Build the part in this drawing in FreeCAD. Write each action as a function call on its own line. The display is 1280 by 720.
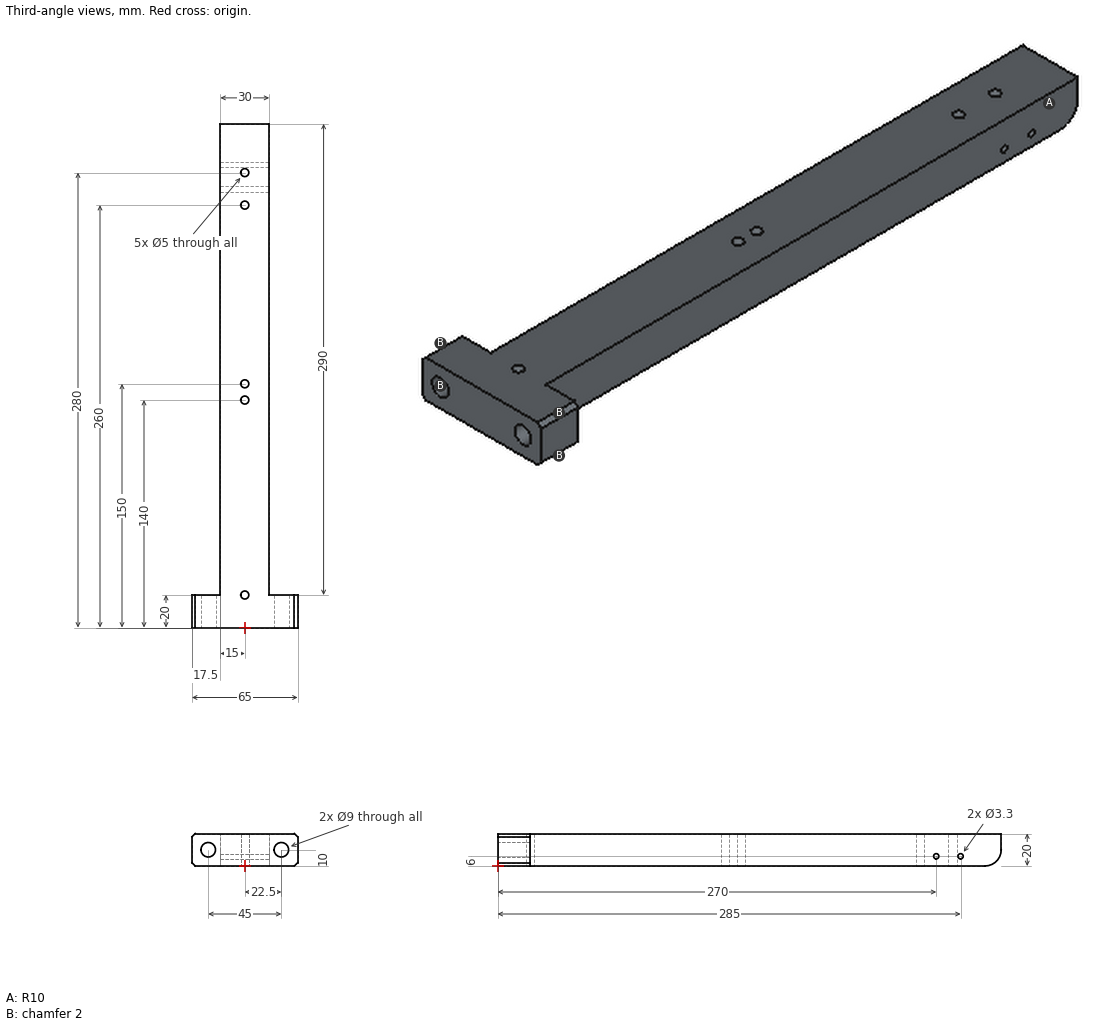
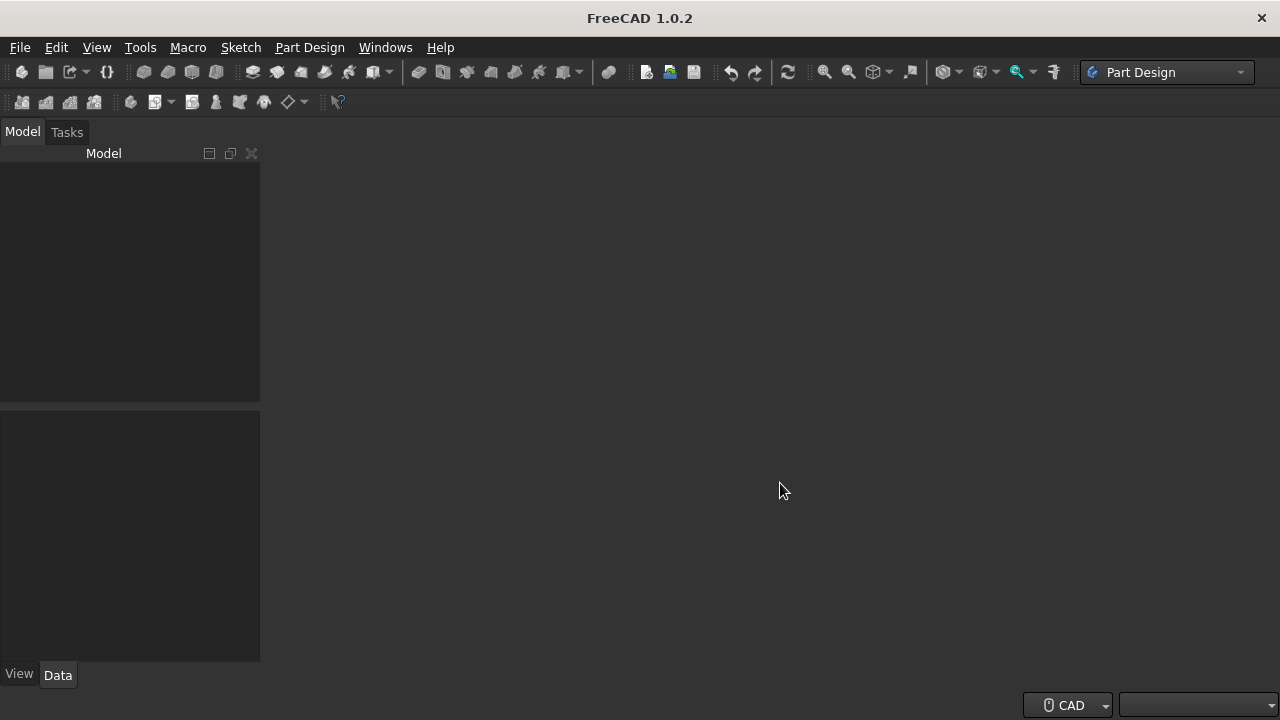
click(646, 72)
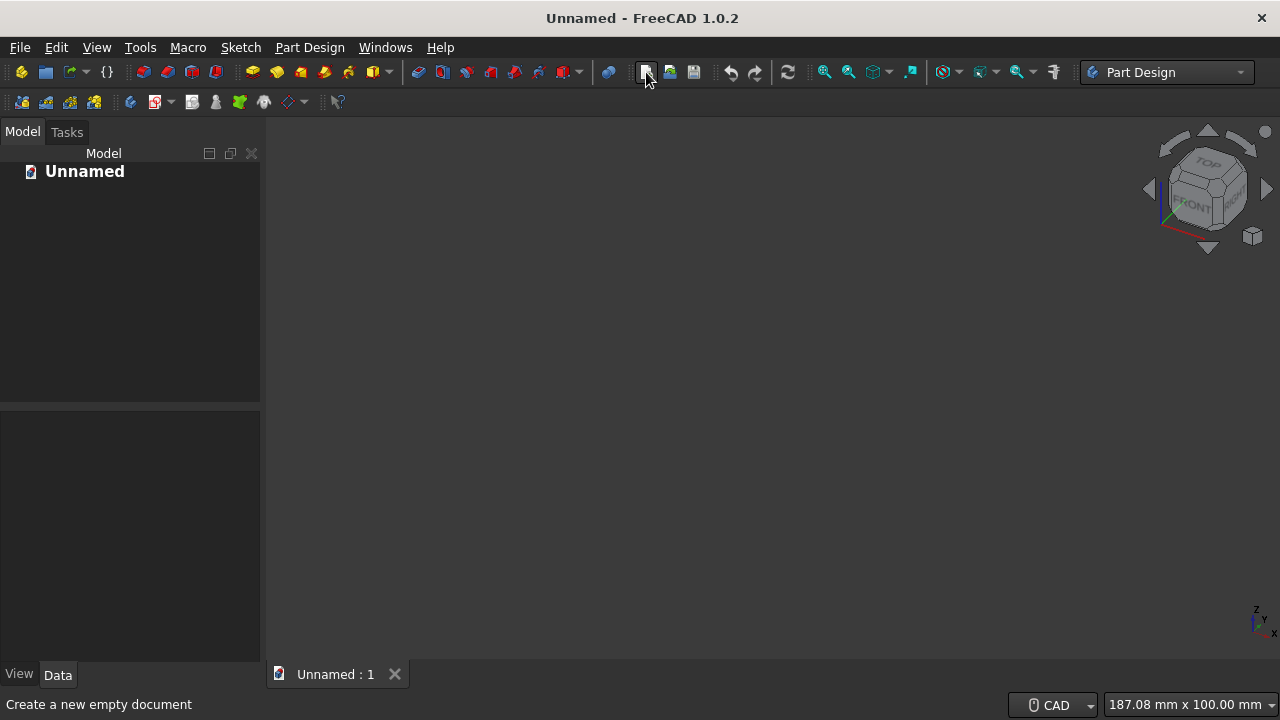
click(156, 102)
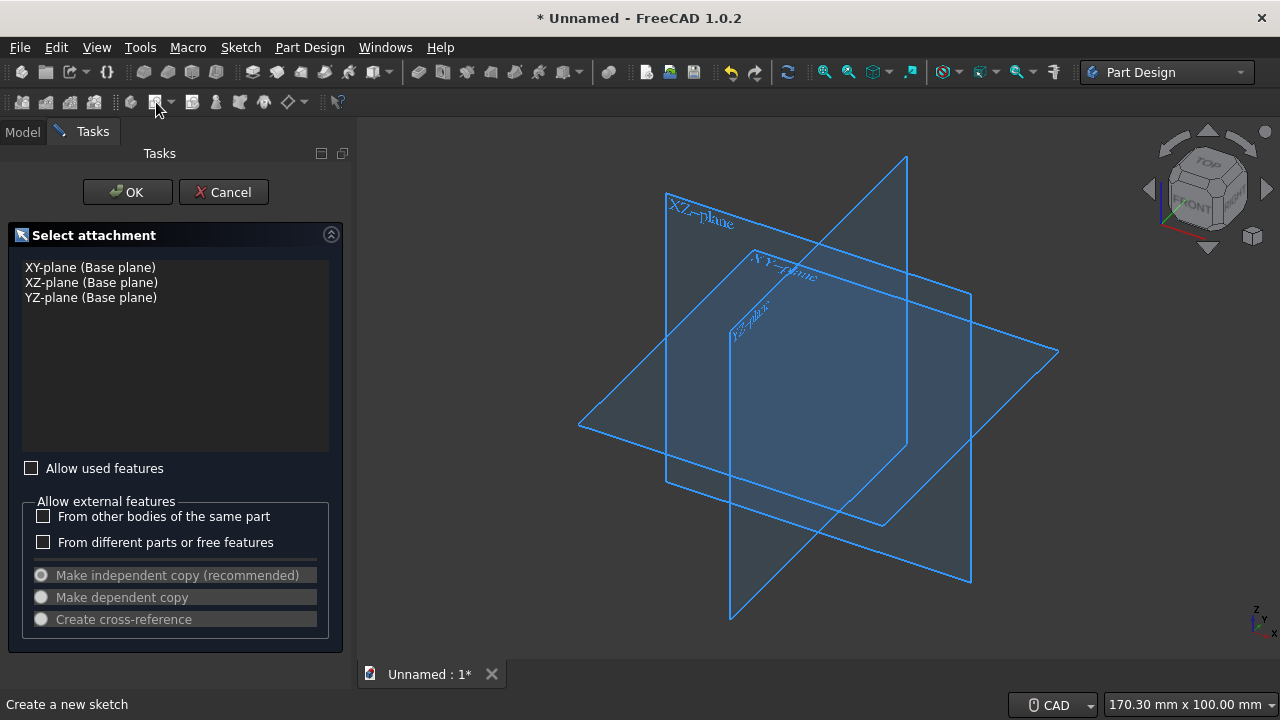
click(82, 268)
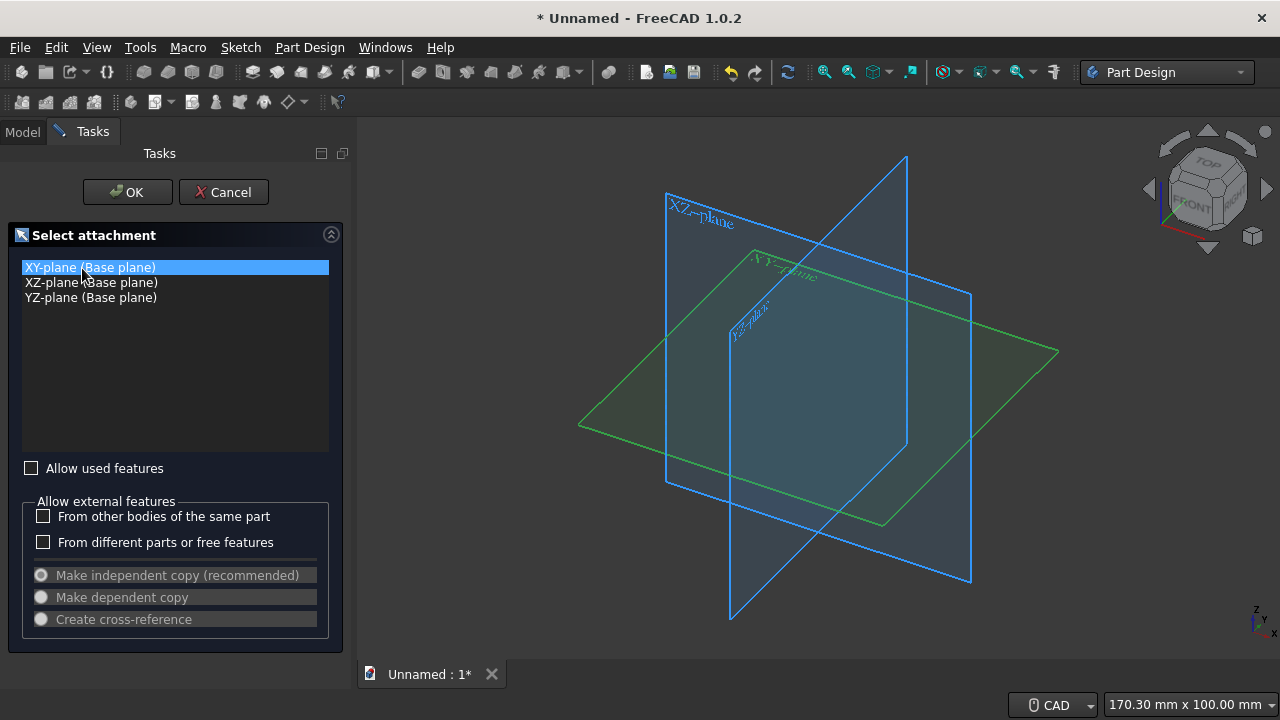
click(128, 192)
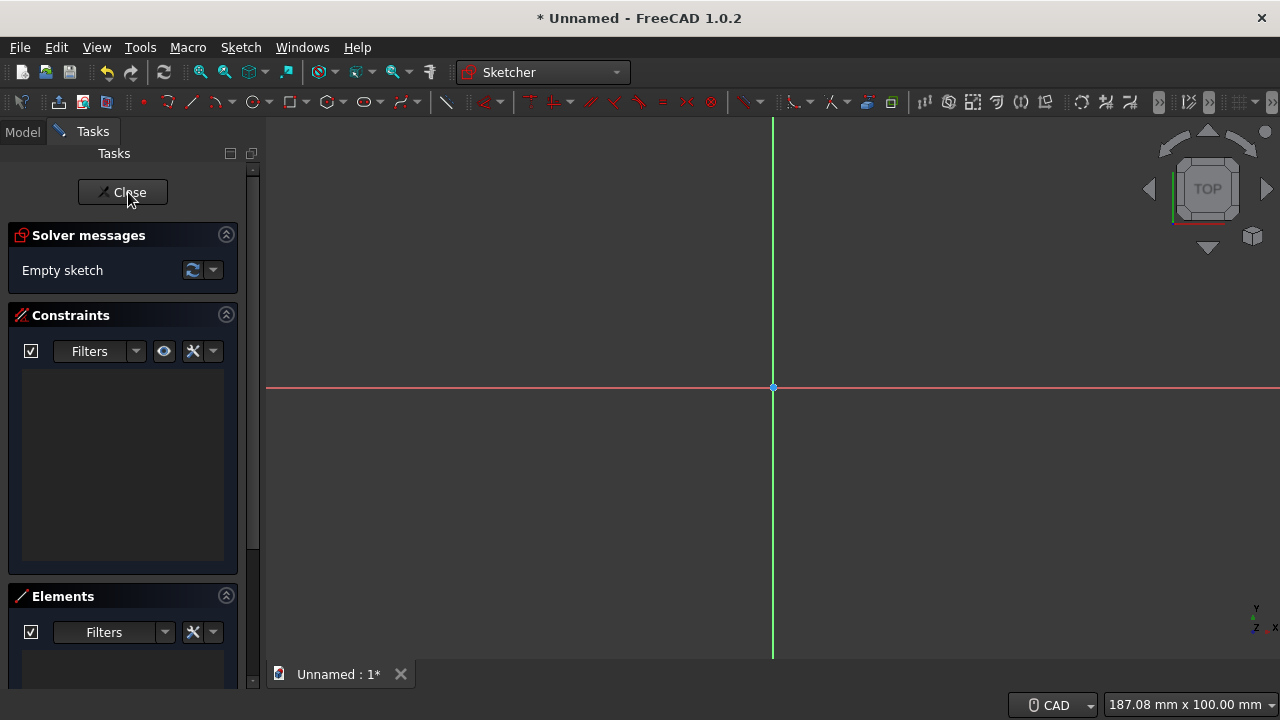
scroll(687, 601, down, 8)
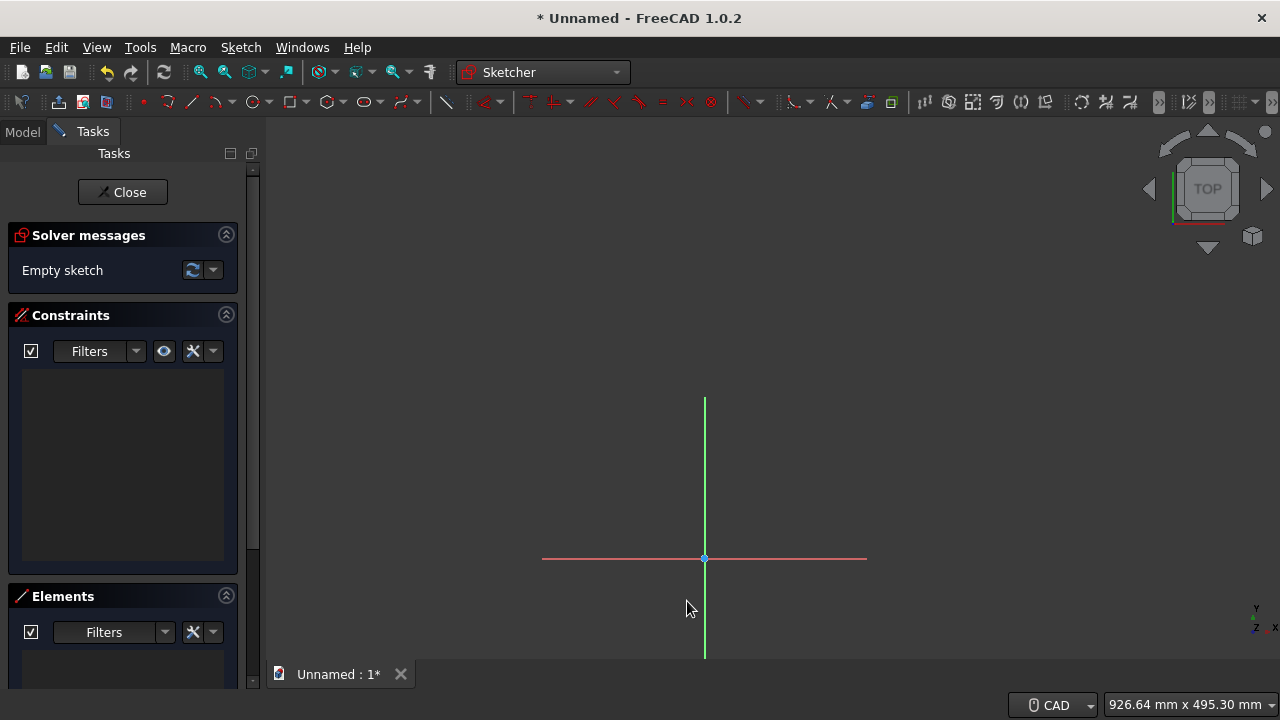
key(g)
key(m)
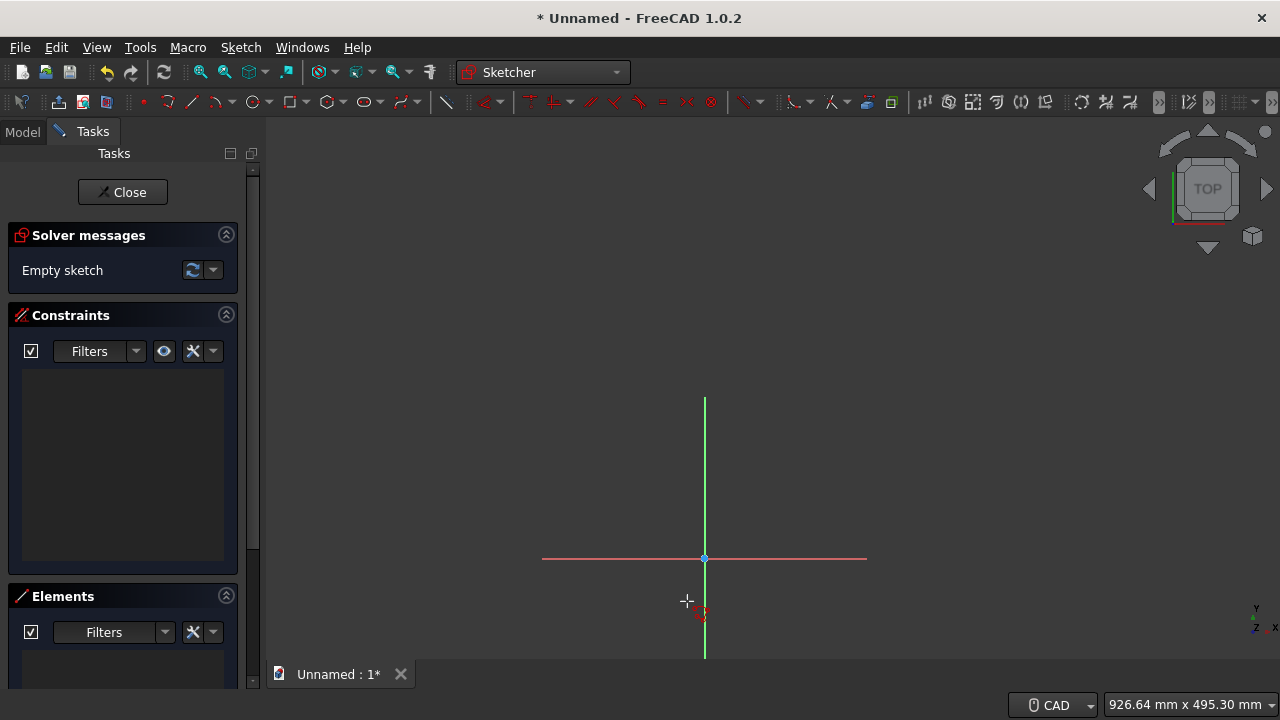
click(688, 537)
click(669, 537)
click(669, 559)
click(740, 550)
click(740, 537)
click(721, 537)
click(721, 219)
click(688, 219)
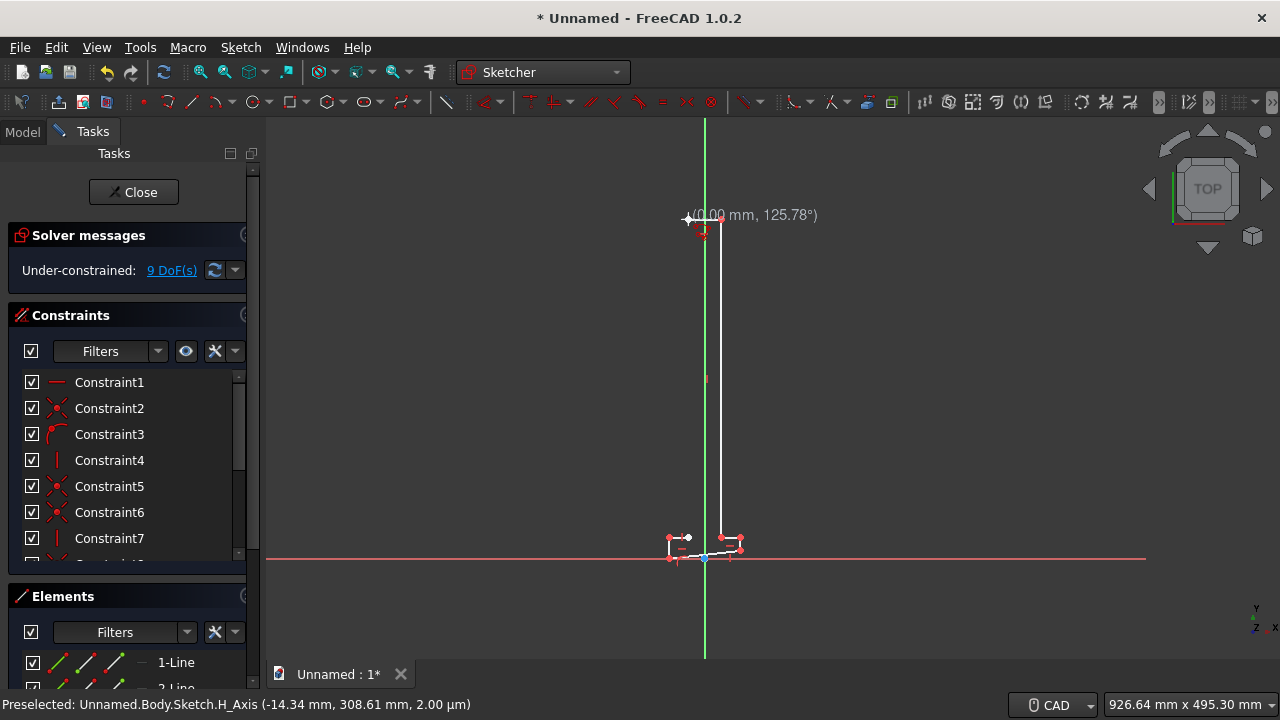
scroll(688, 537, up, 3)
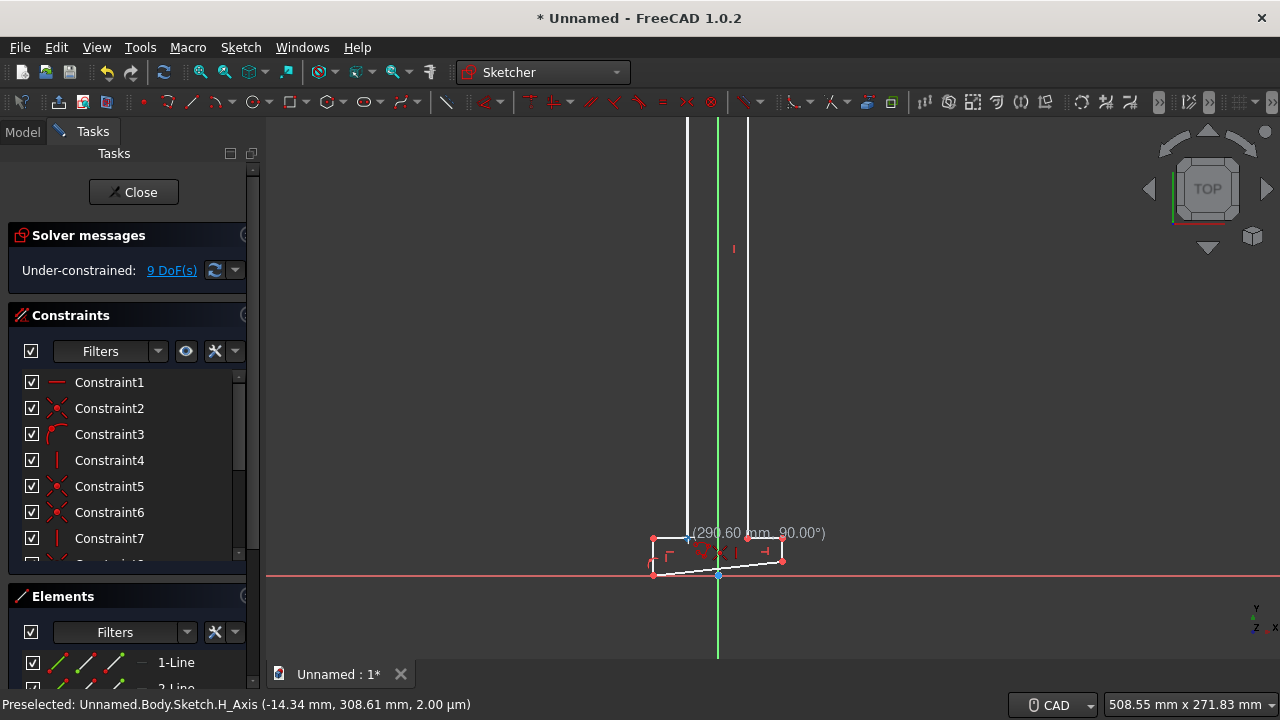
click(688, 538)
key(Escape)
key(Escape)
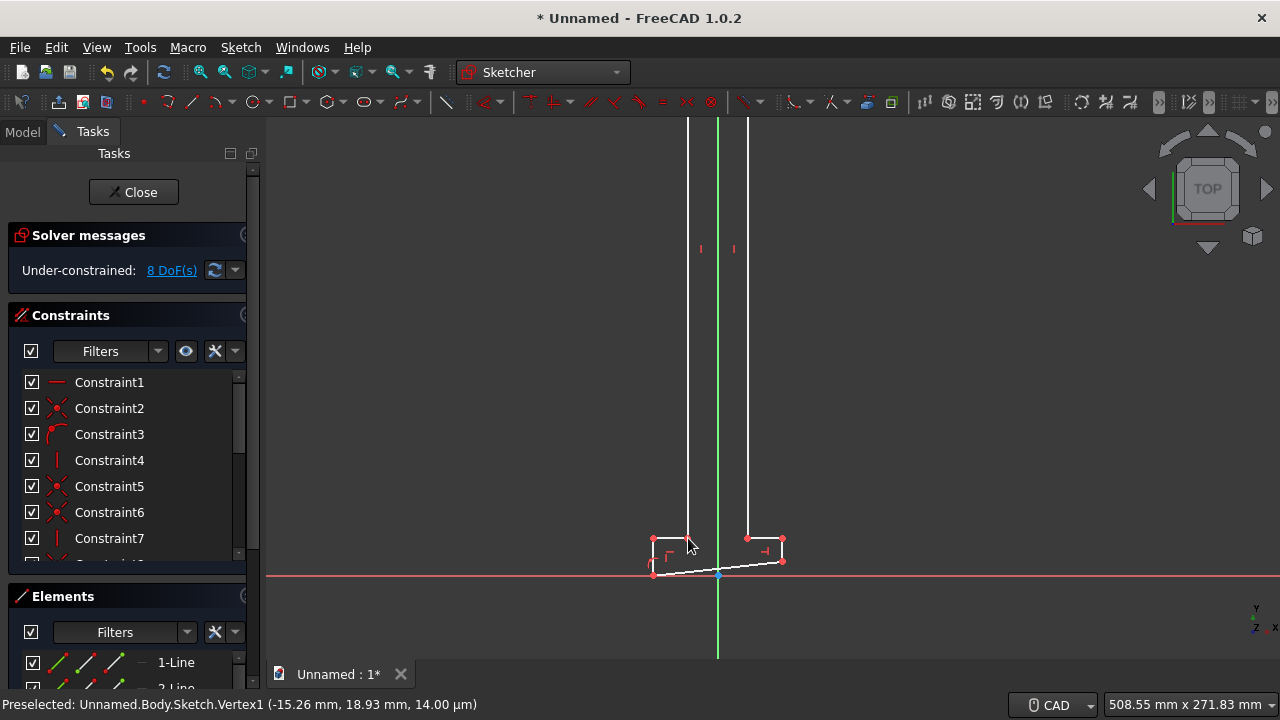
scroll(744, 566, up, 2)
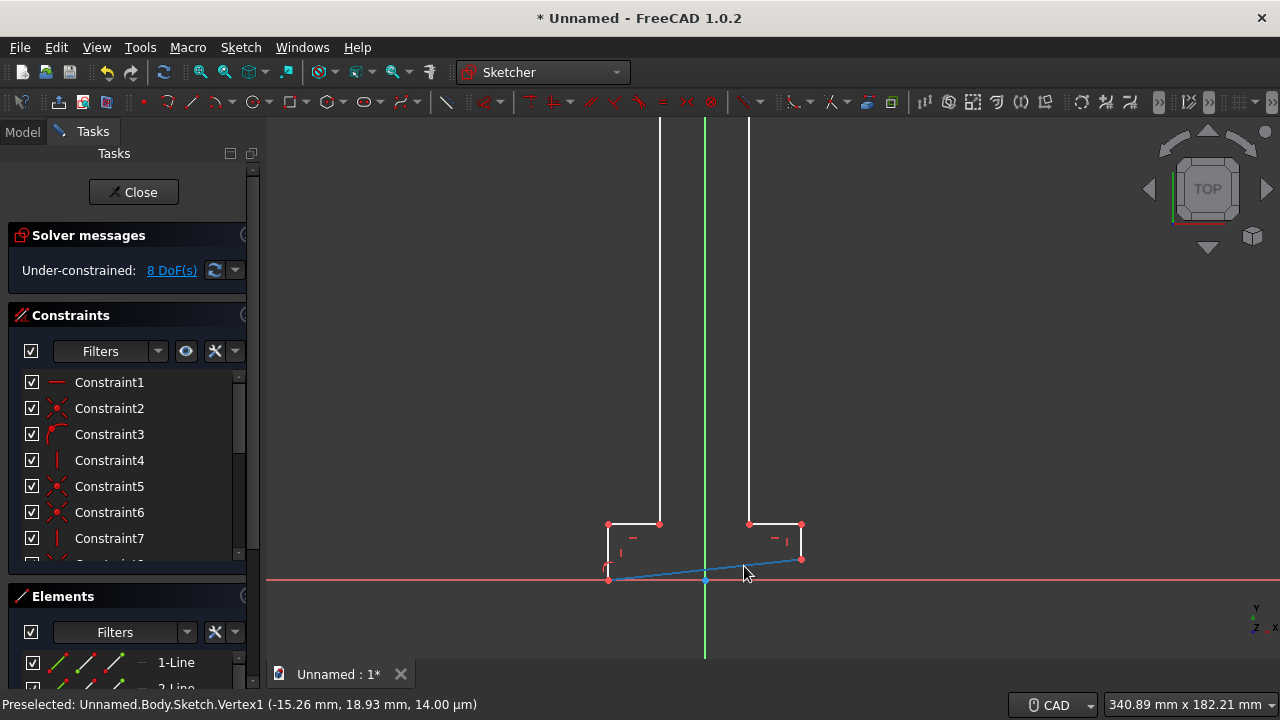
click(743, 566)